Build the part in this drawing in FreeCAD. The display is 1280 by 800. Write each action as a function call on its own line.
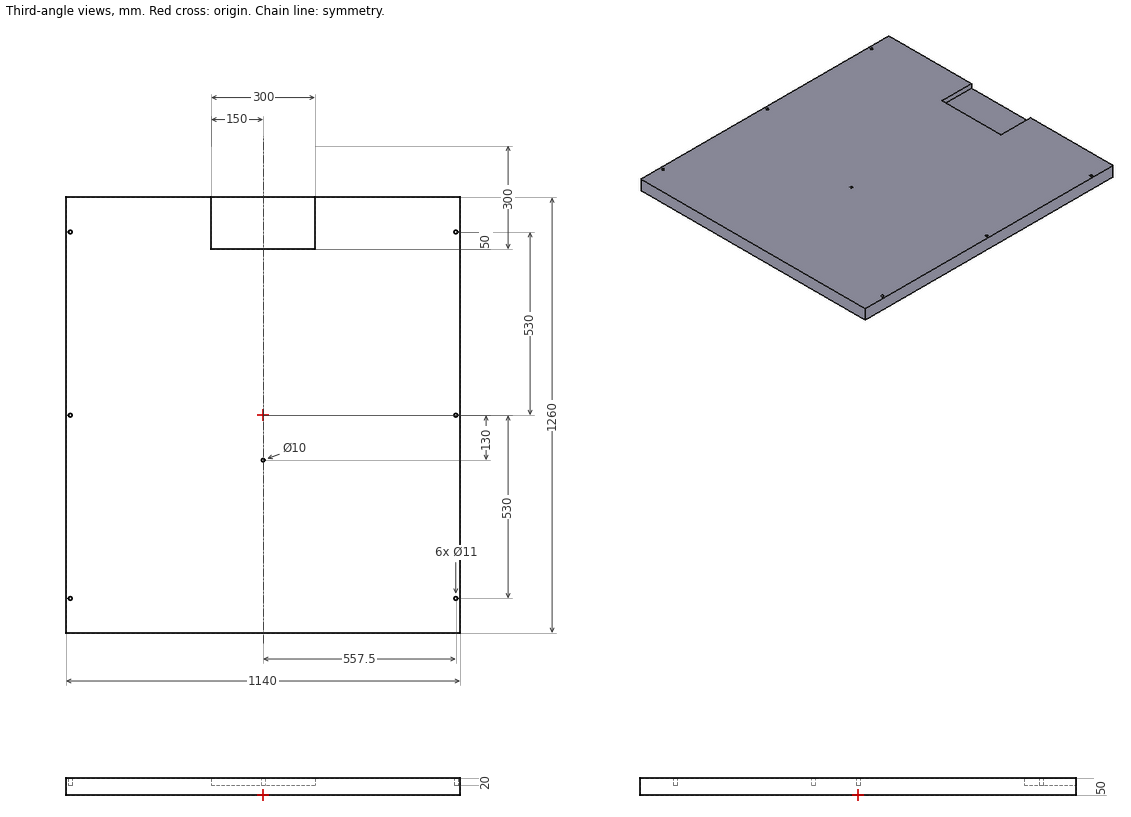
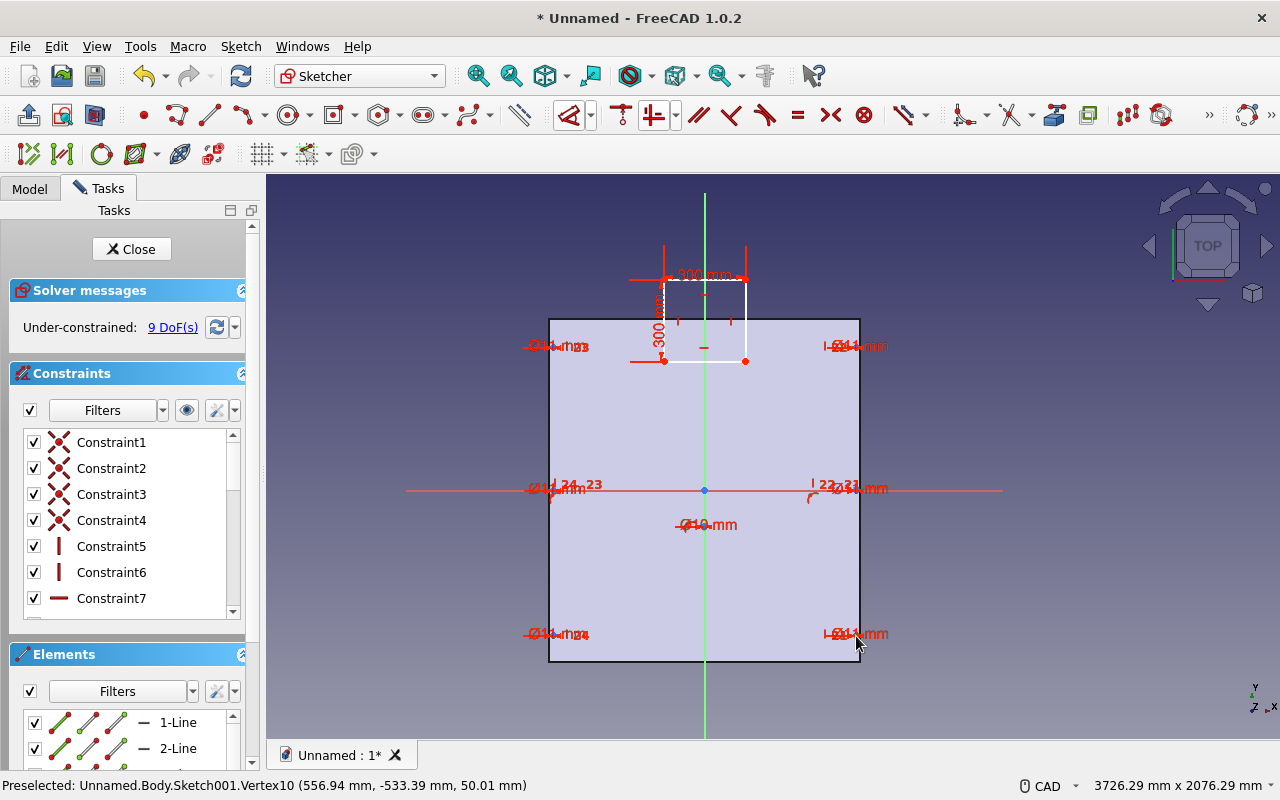
click(553, 636)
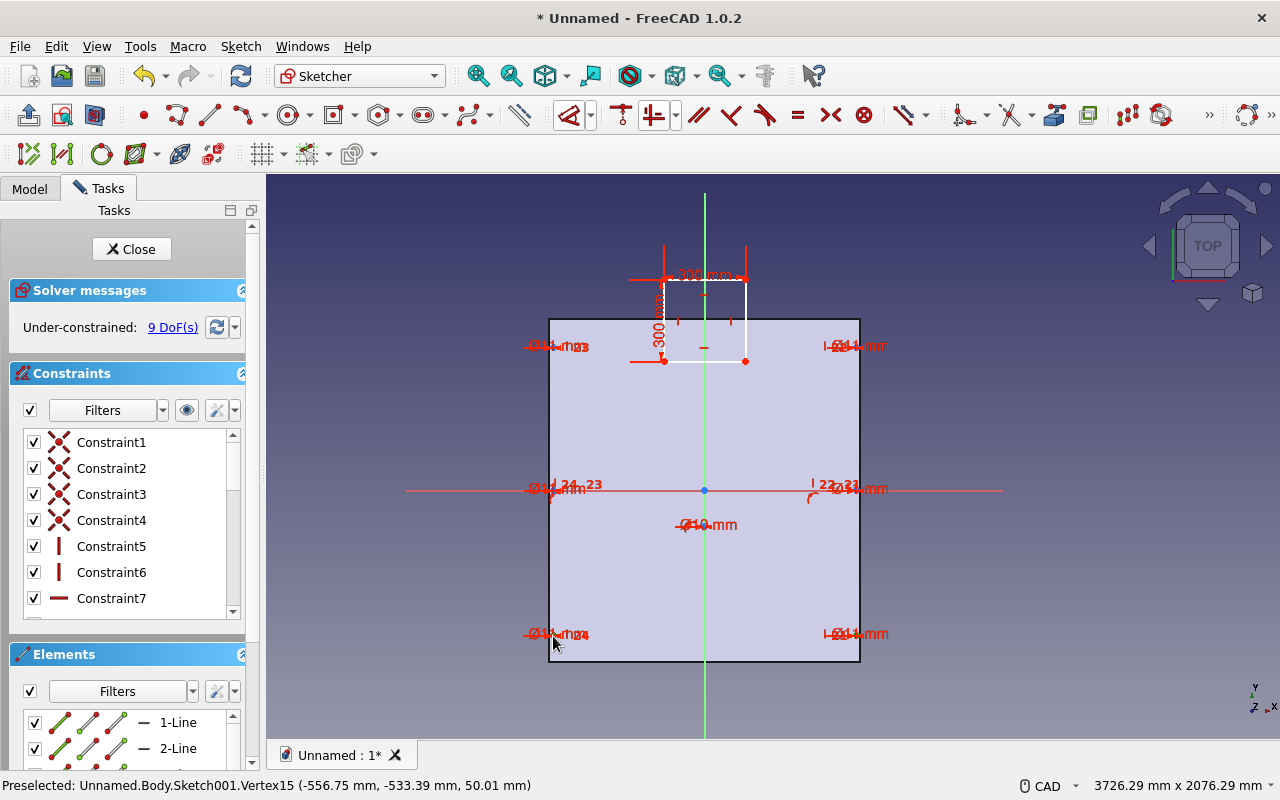
key(h)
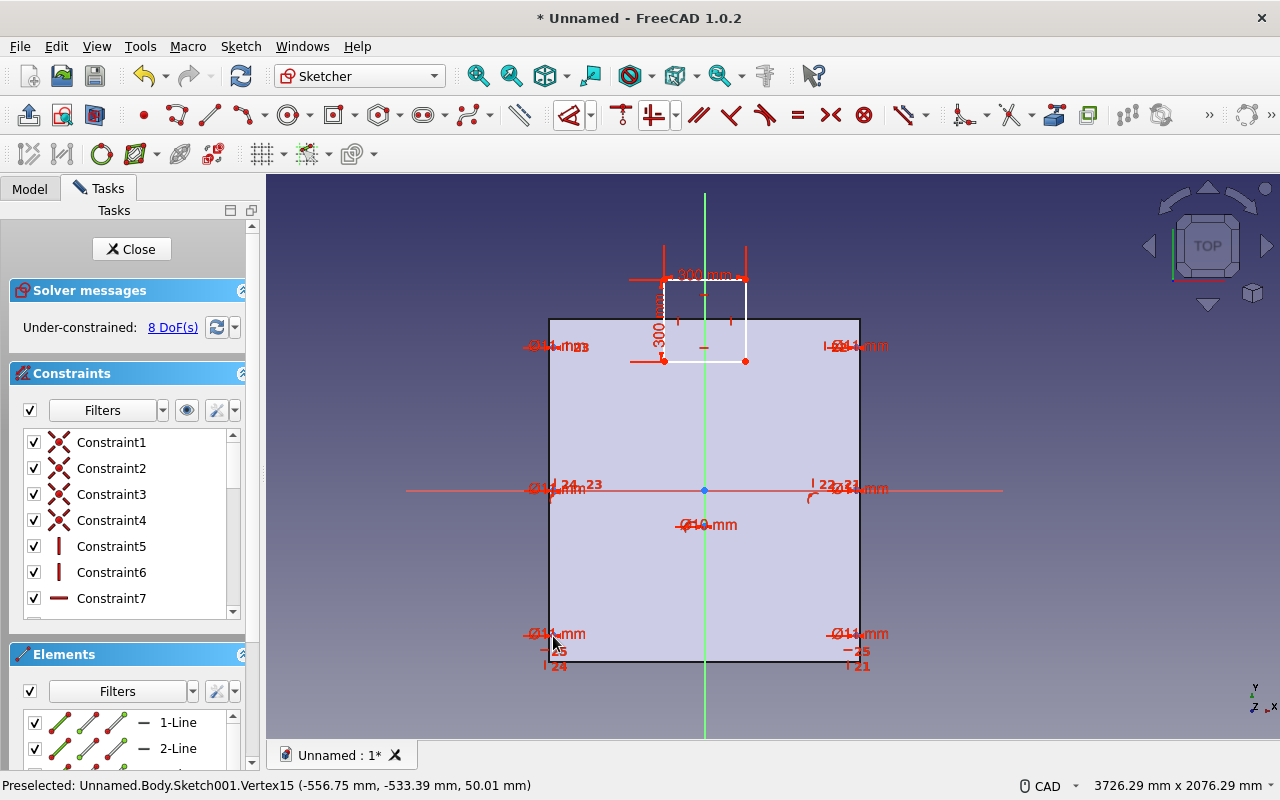
click(856, 348)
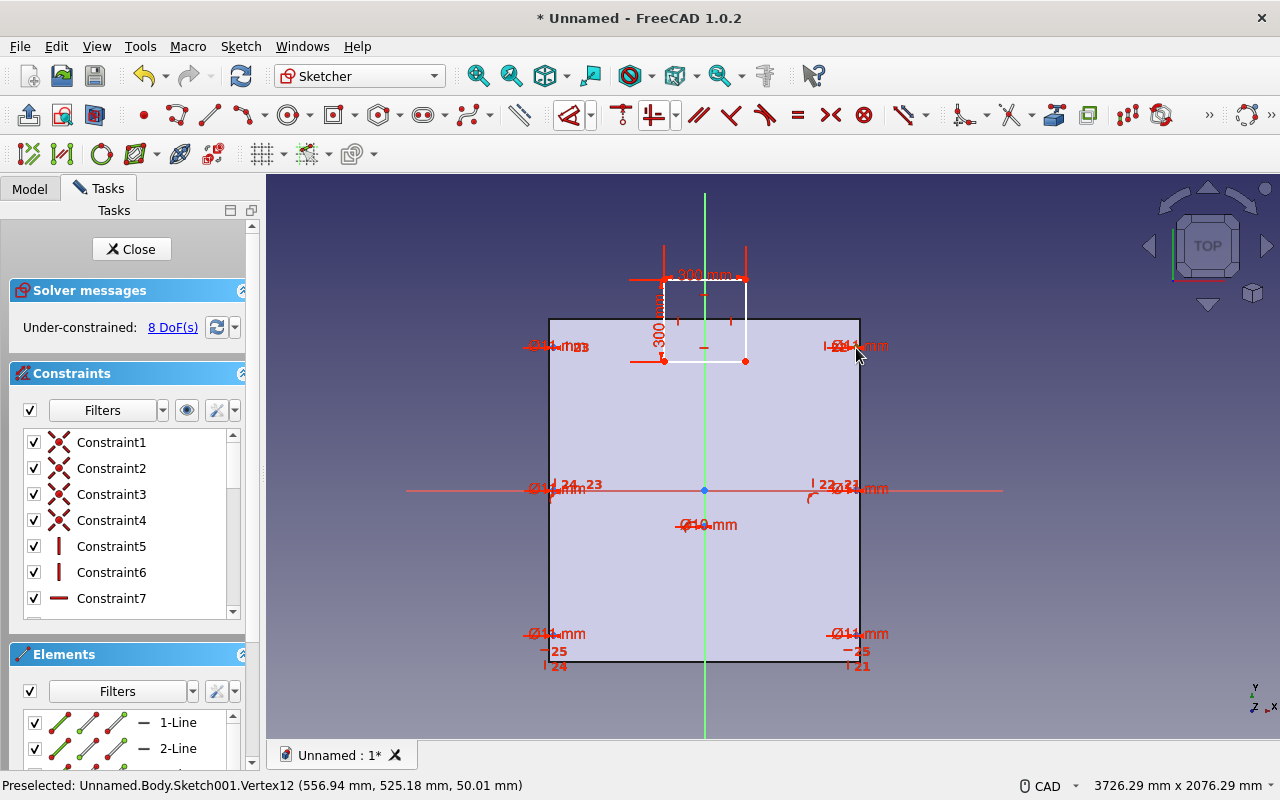
click(553, 348)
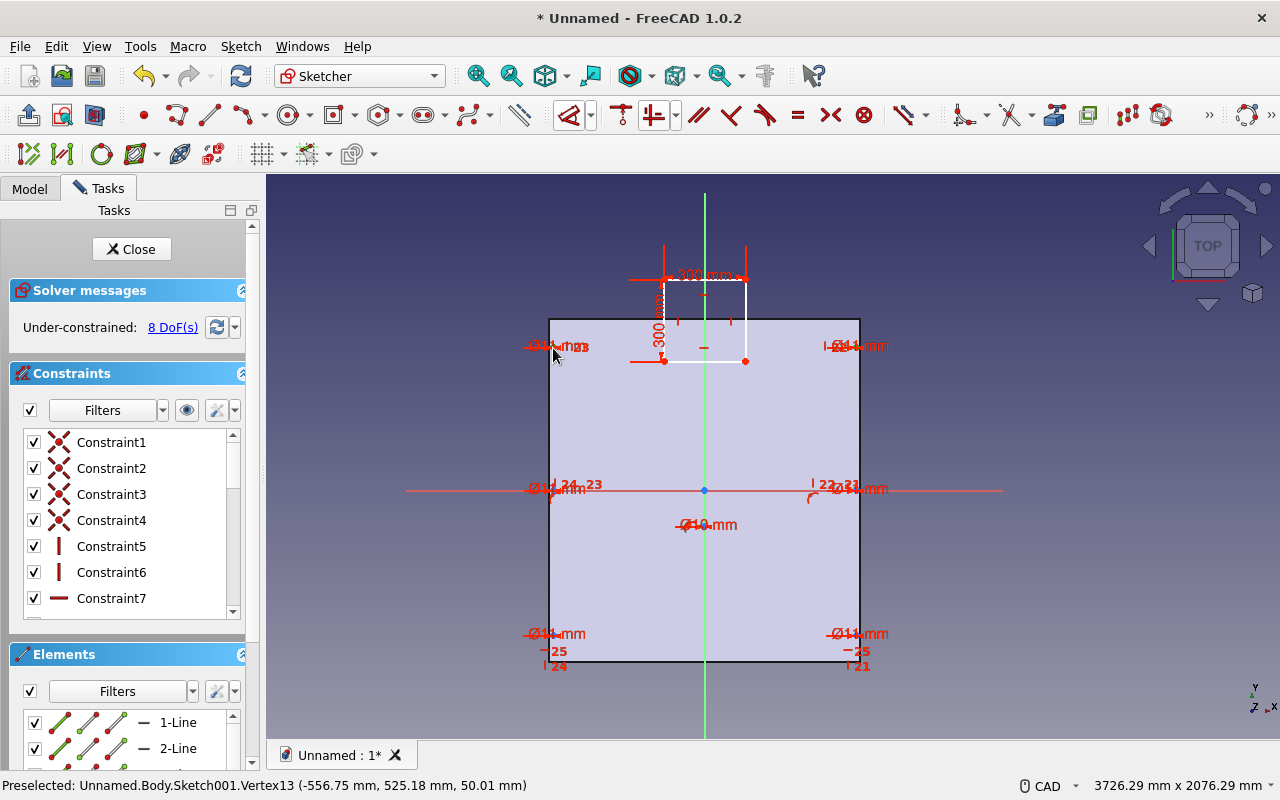
click(705, 675)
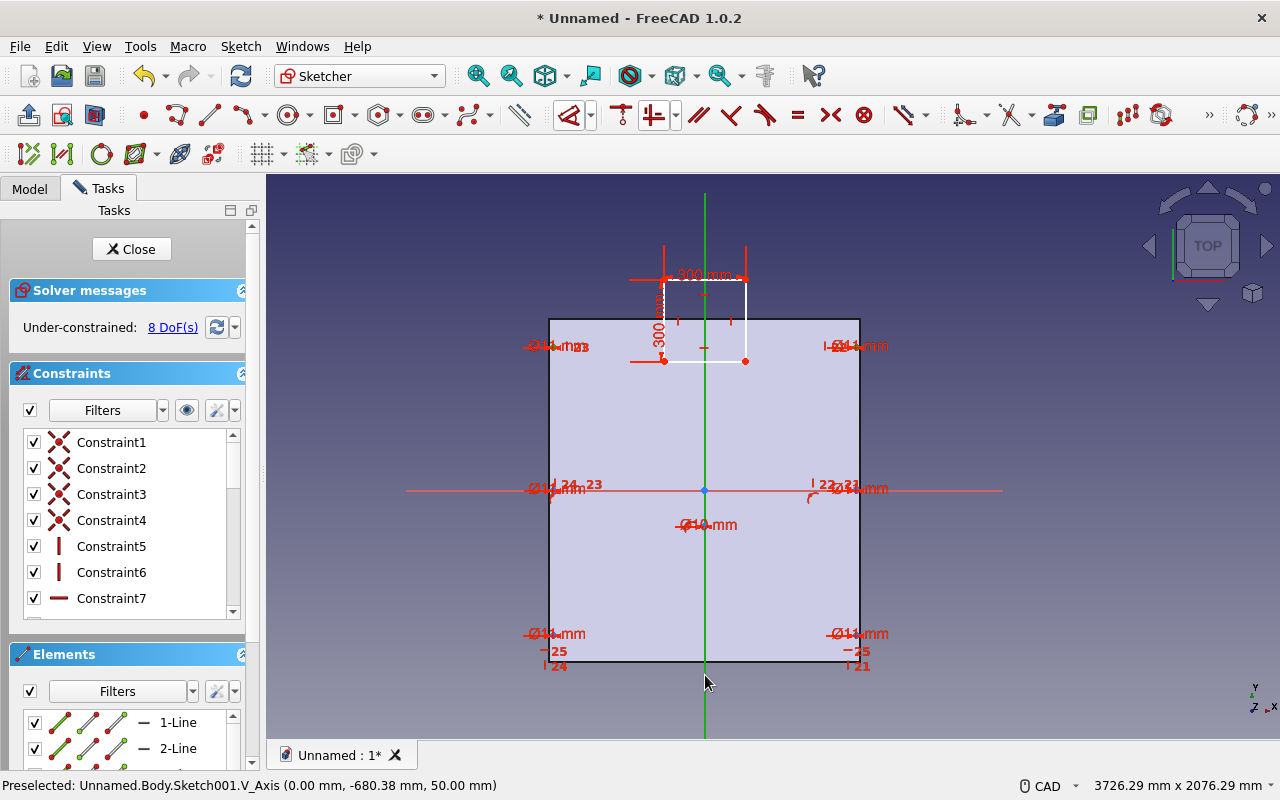
click(831, 116)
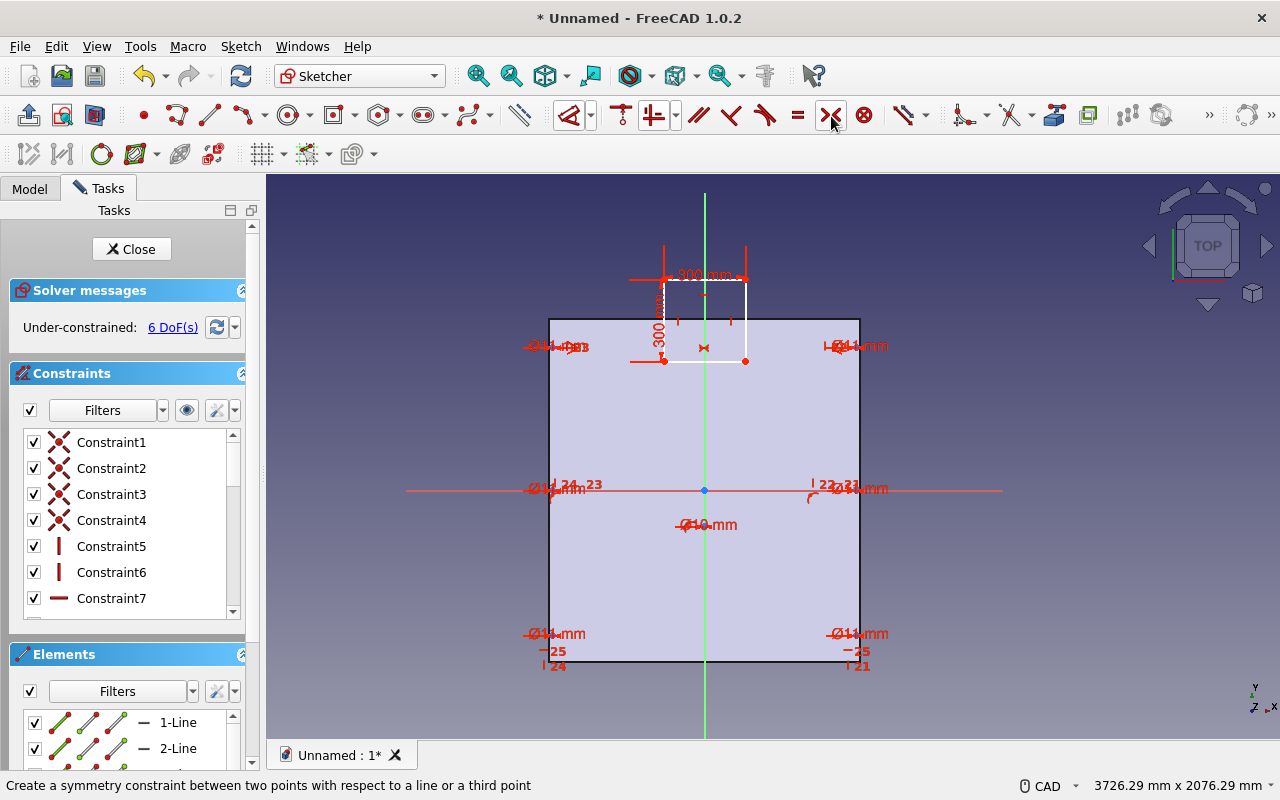
click(705, 527)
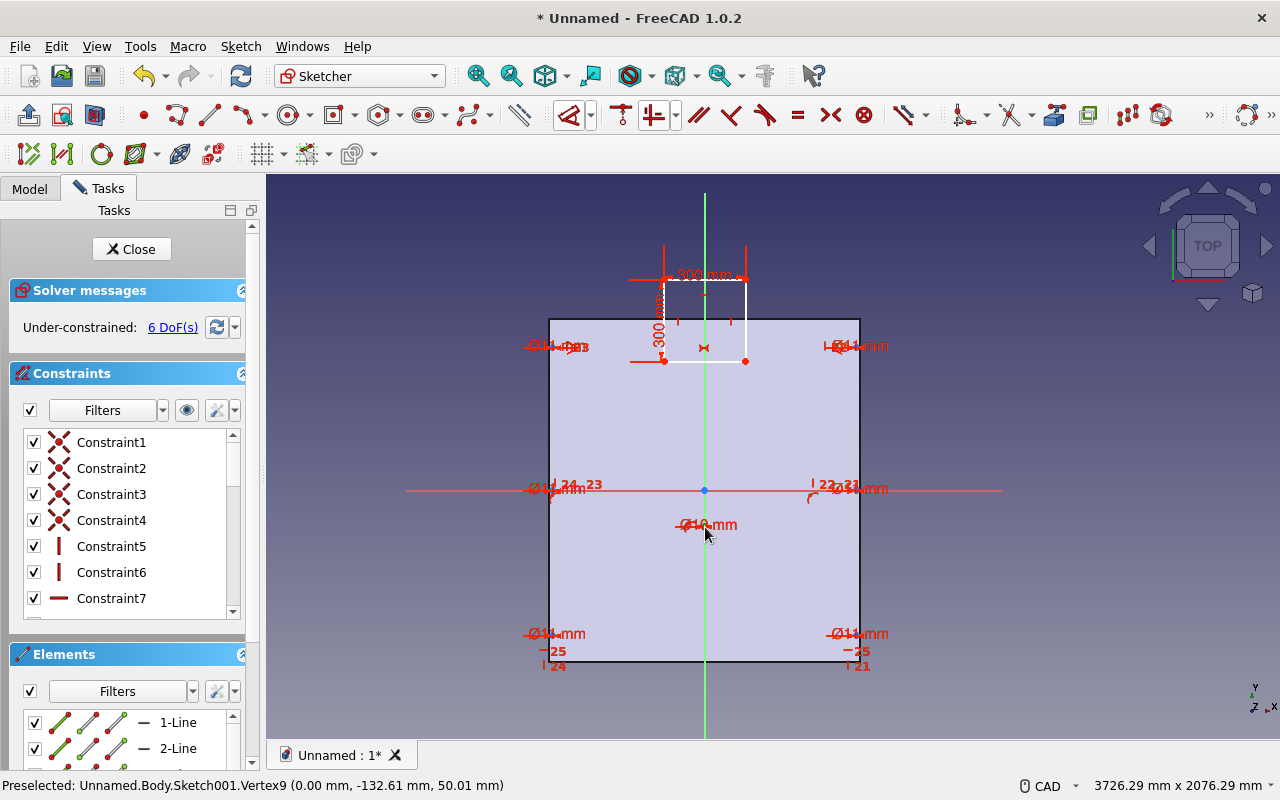
key(i)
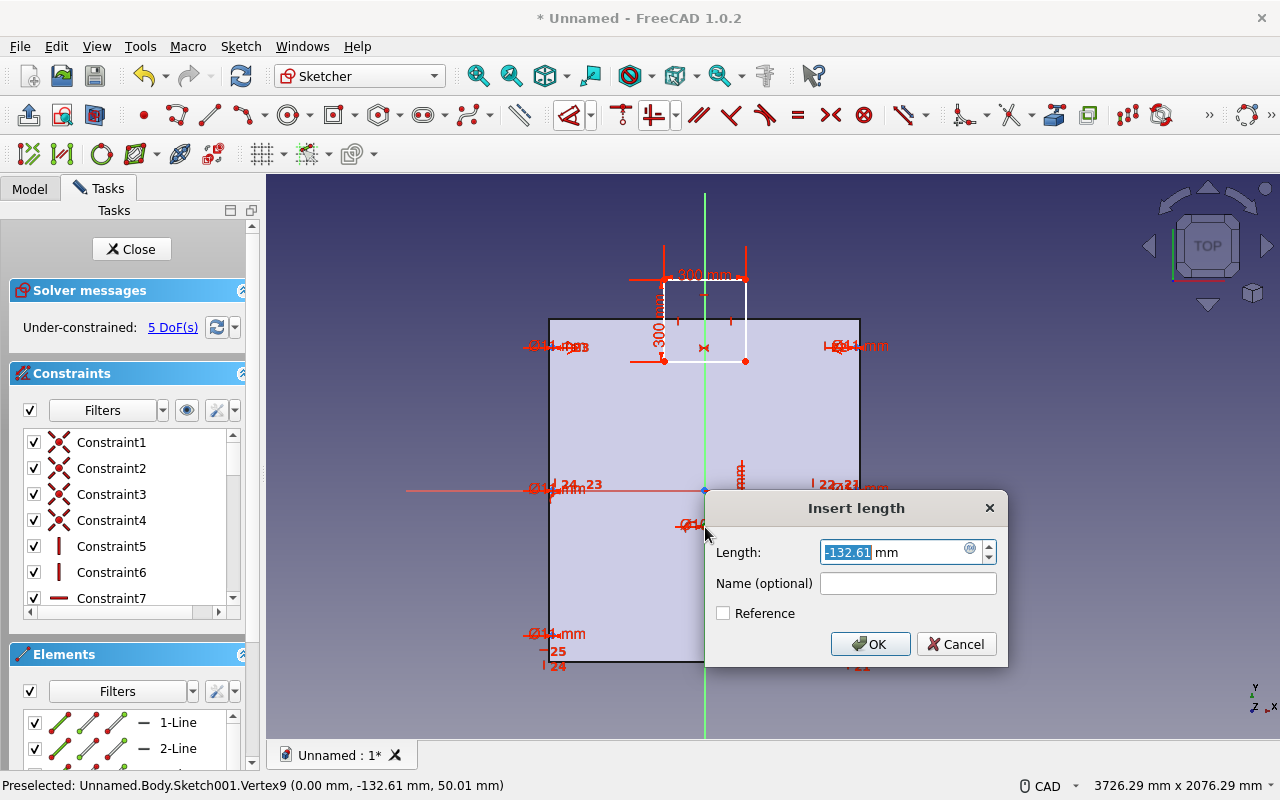
text(-130)
key(Return)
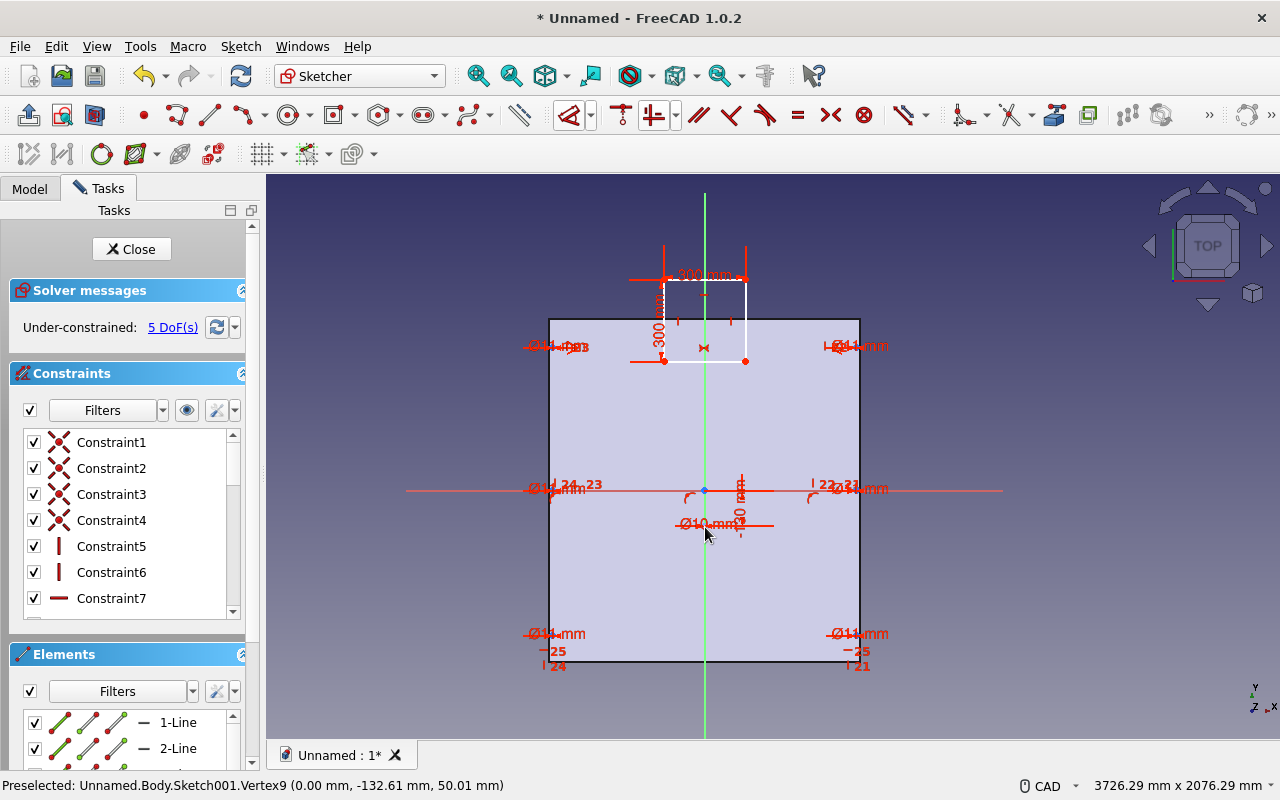
click(856, 636)